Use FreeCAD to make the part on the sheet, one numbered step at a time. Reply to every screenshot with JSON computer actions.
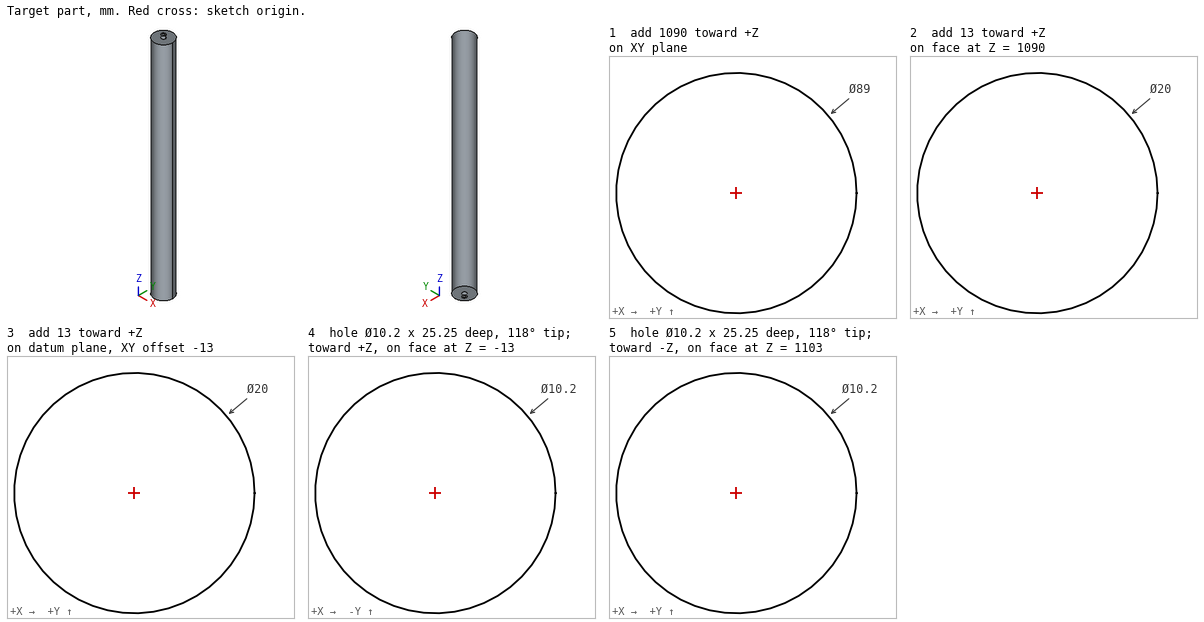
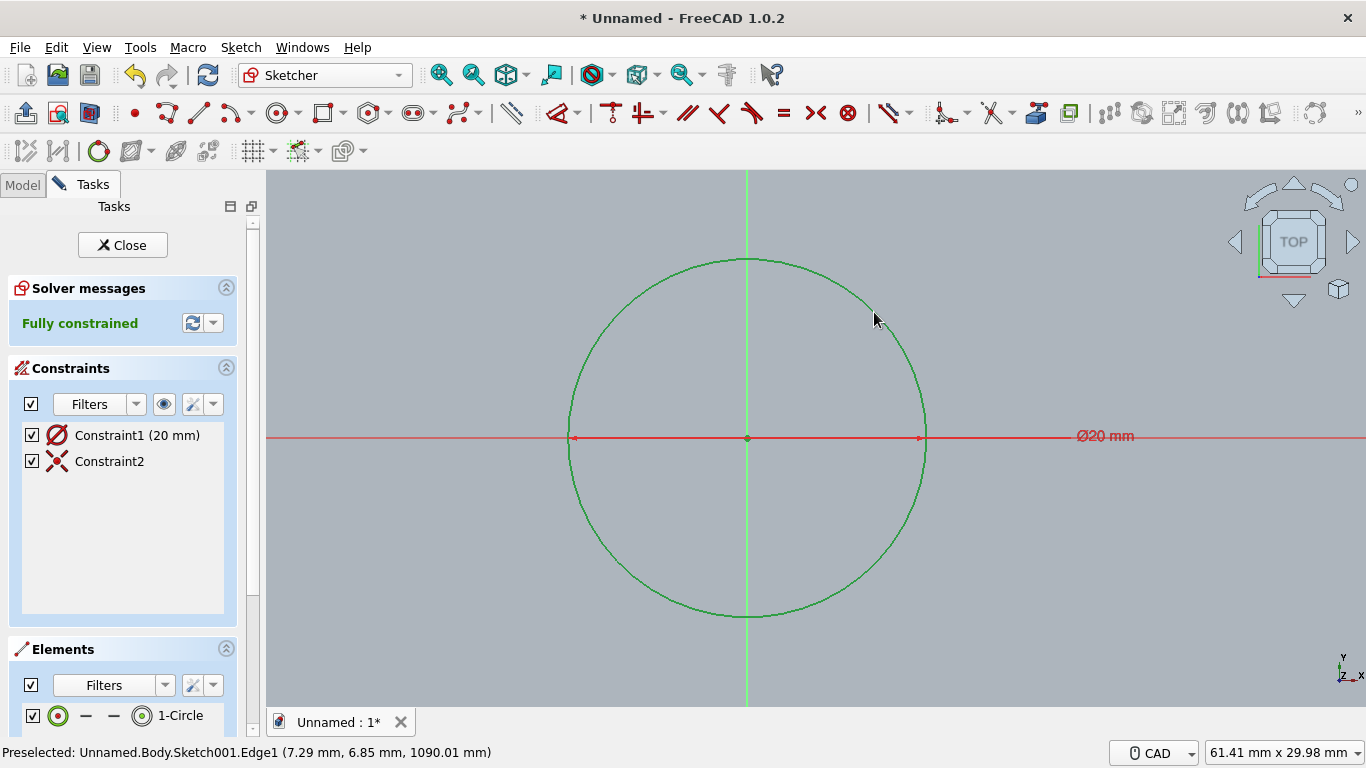
{"action": "left_click", "coordinate": [123, 245]}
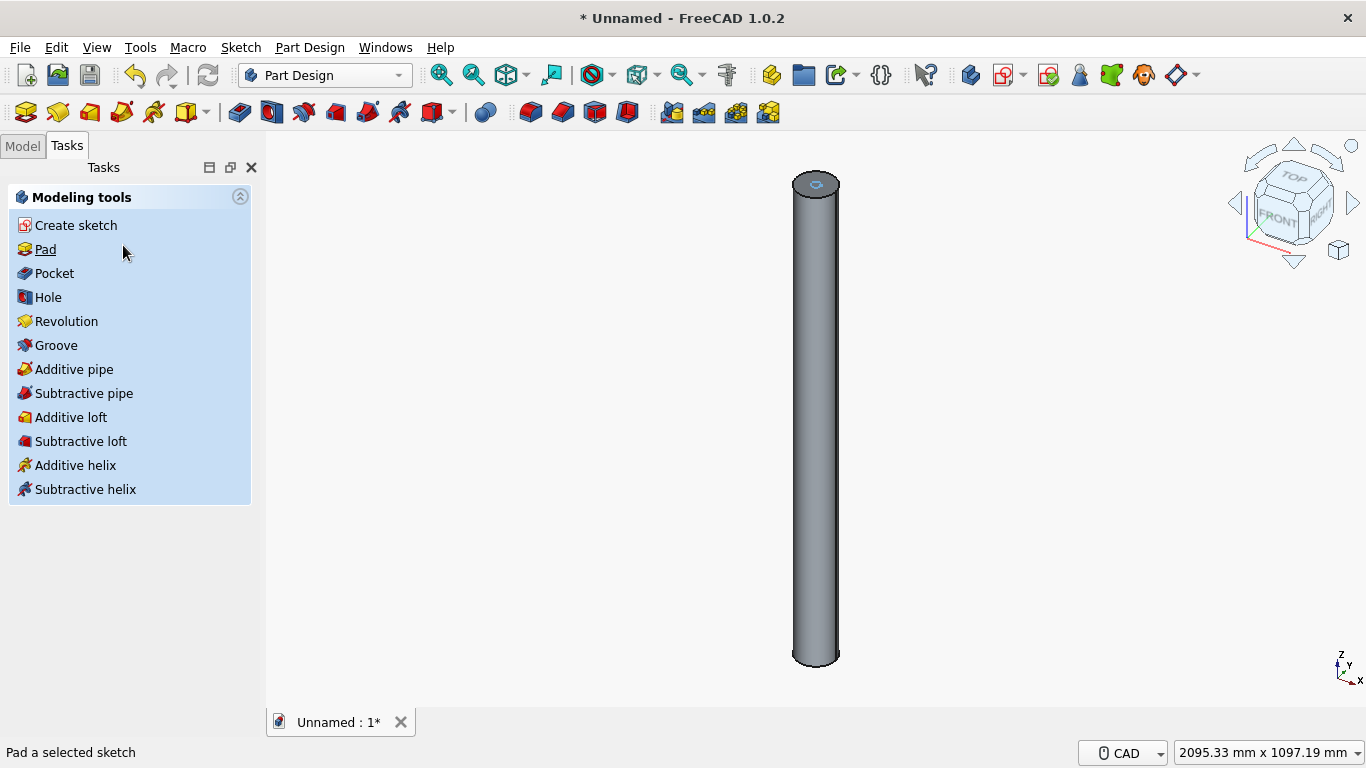
{"action": "left_click", "coordinate": [26, 112]}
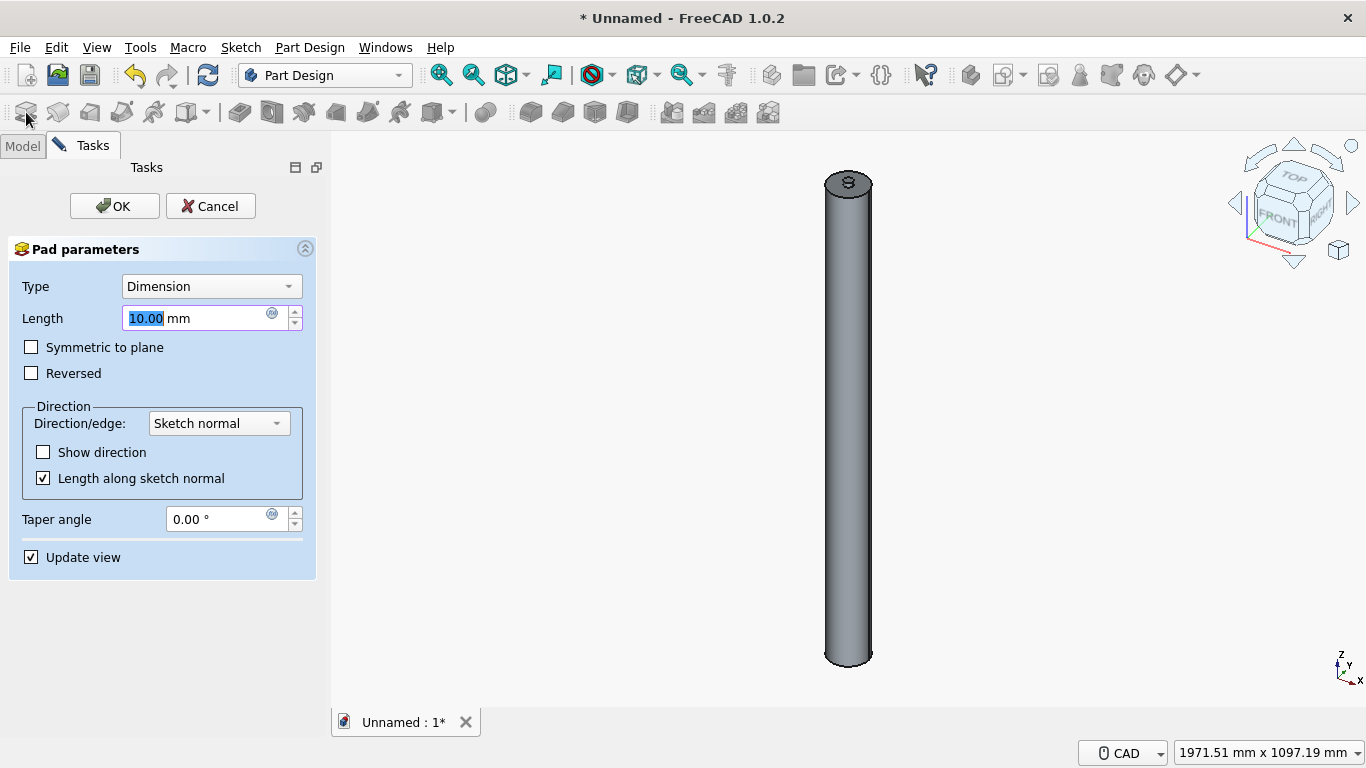
{"action": "type", "text": "13"}
{"action": "key", "text": "Tab"}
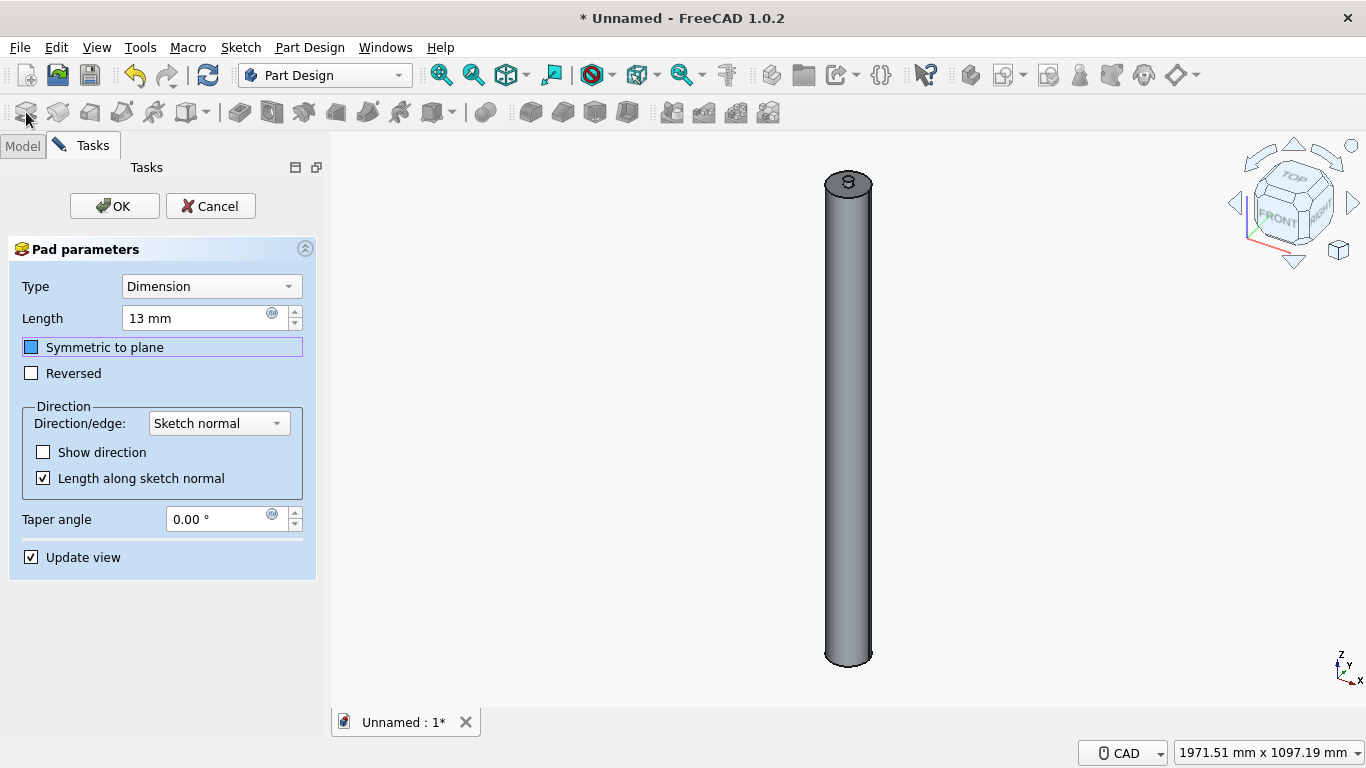
{"action": "left_click", "coordinate": [115, 206]}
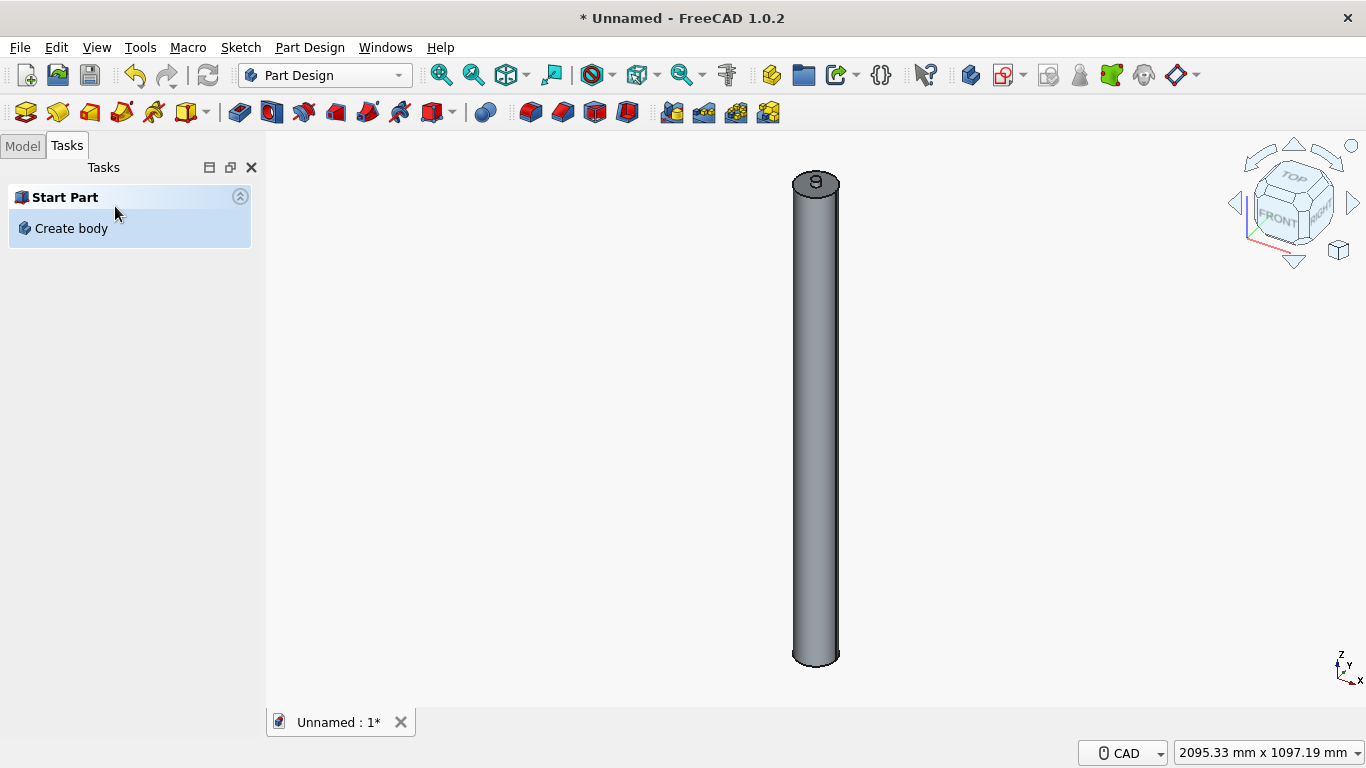
{"action": "left_click", "coordinate": [23, 145]}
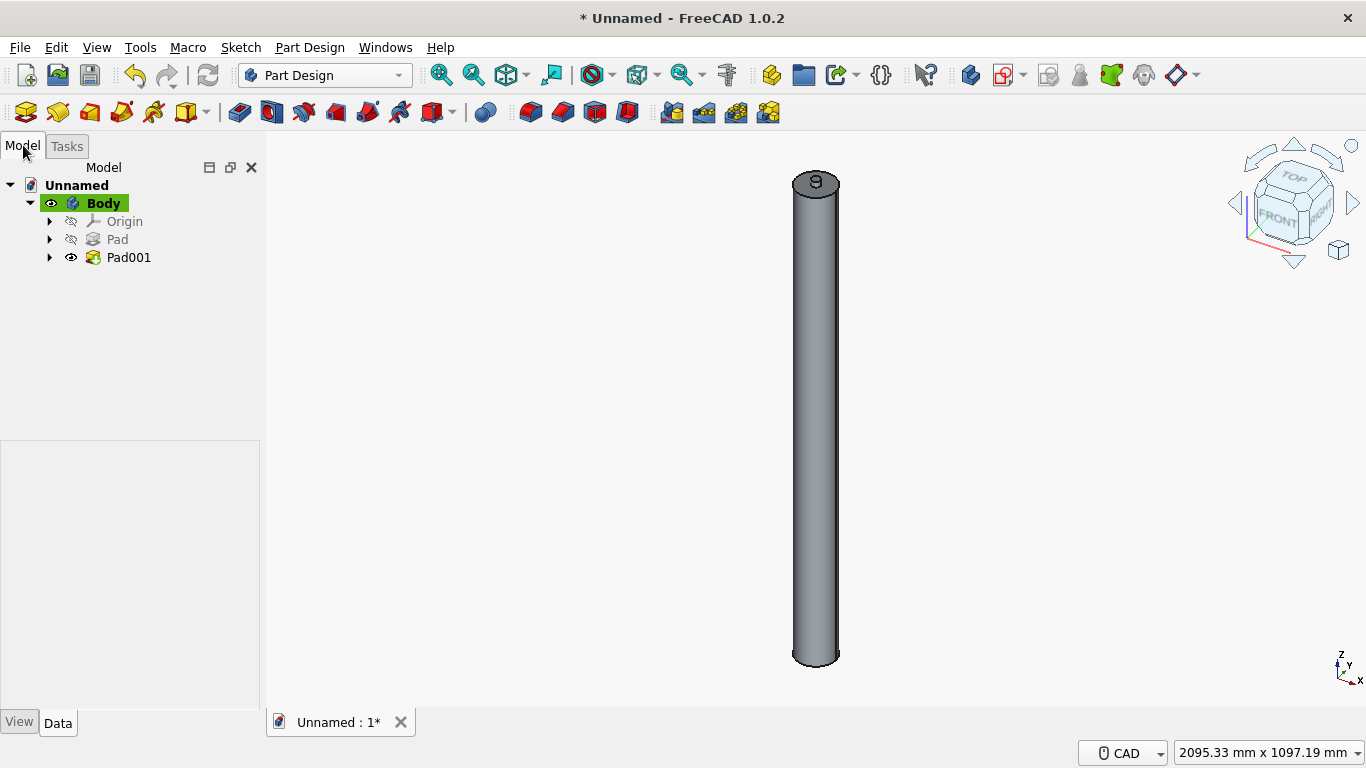
{"action": "left_click", "coordinate": [50, 221]}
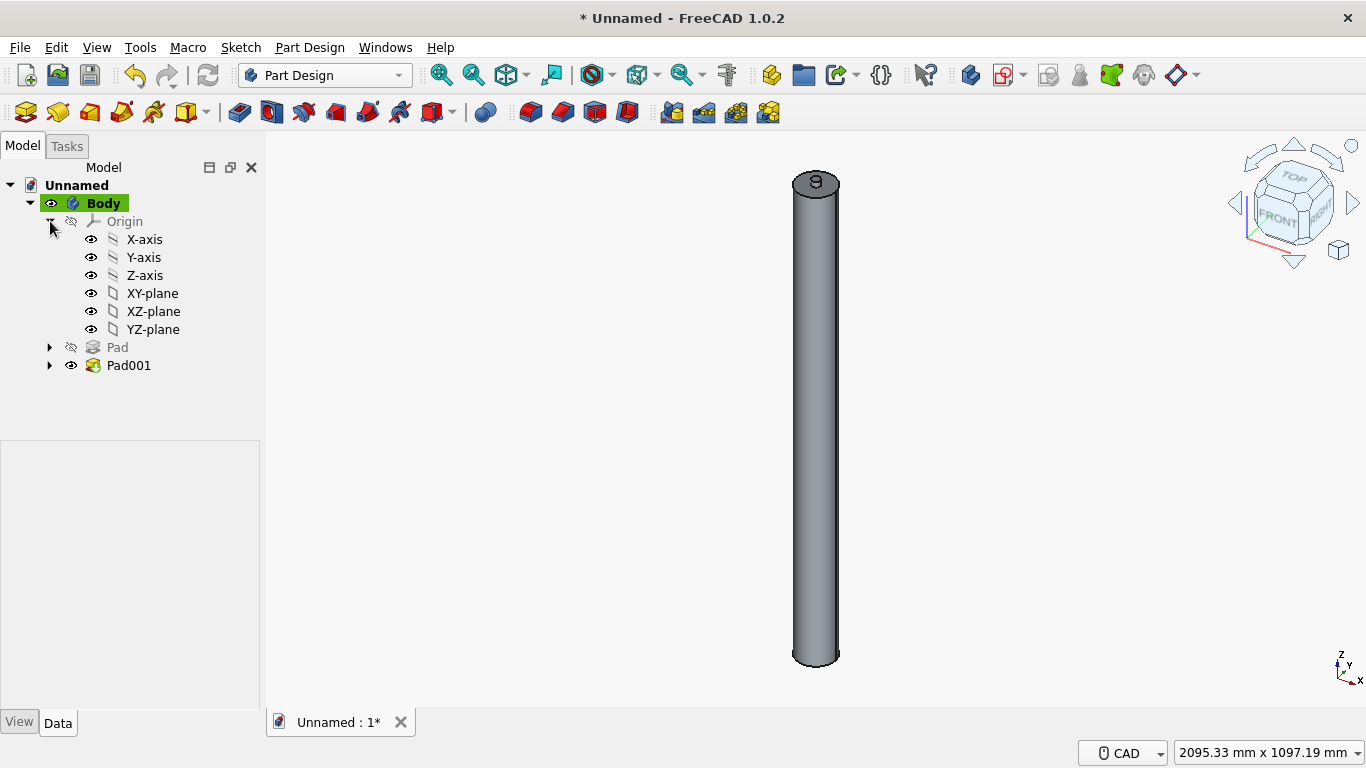
{"action": "left_click", "coordinate": [136, 293]}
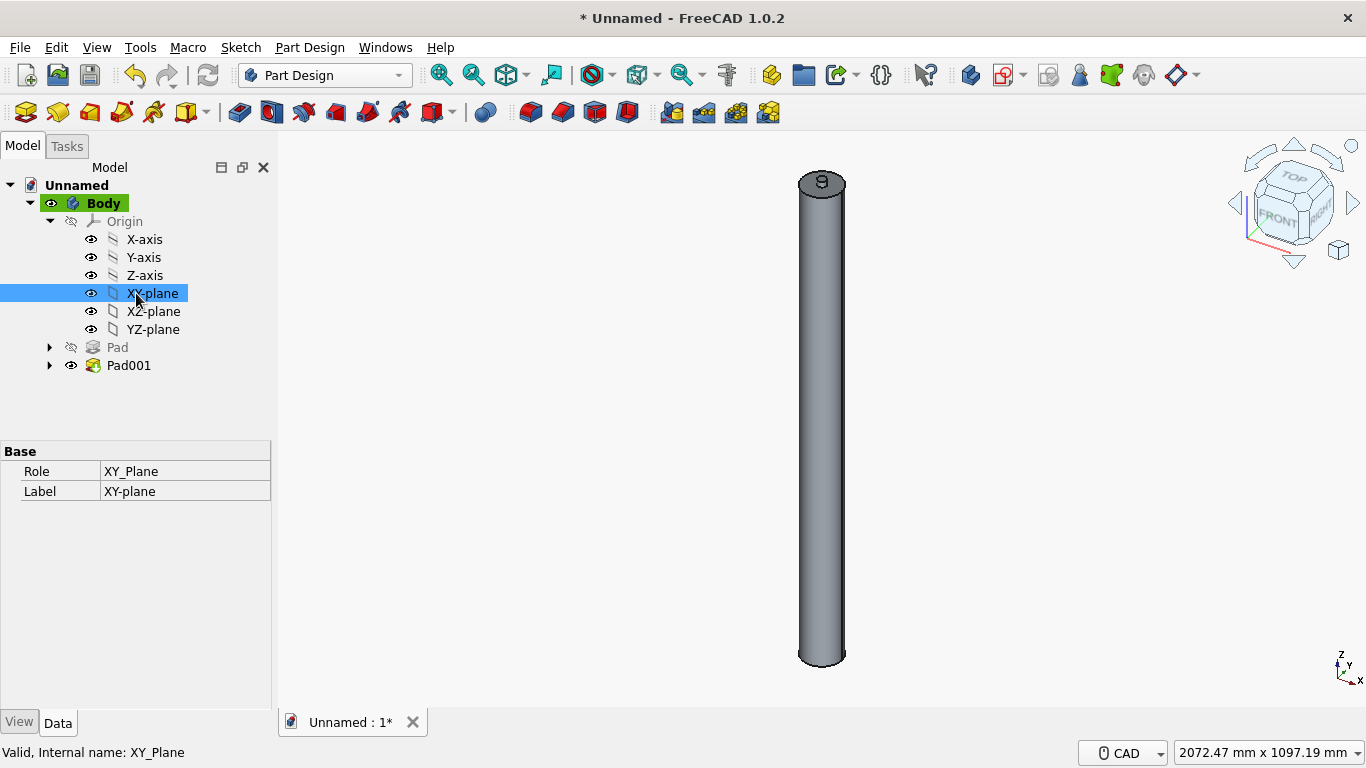
{"action": "left_click", "coordinate": [1176, 76]}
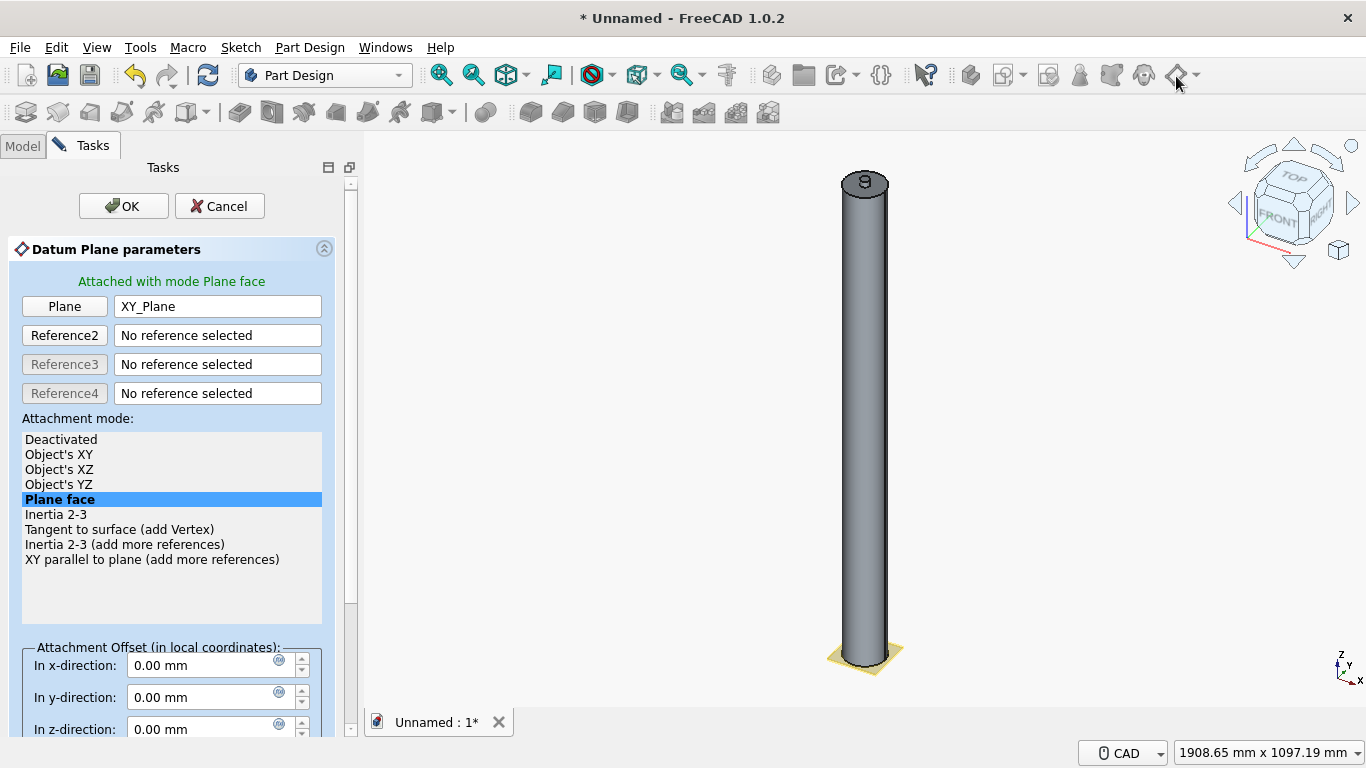
{"action": "scroll", "coordinate": [351, 456], "scroll_direction": "down", "scroll_amount": 2}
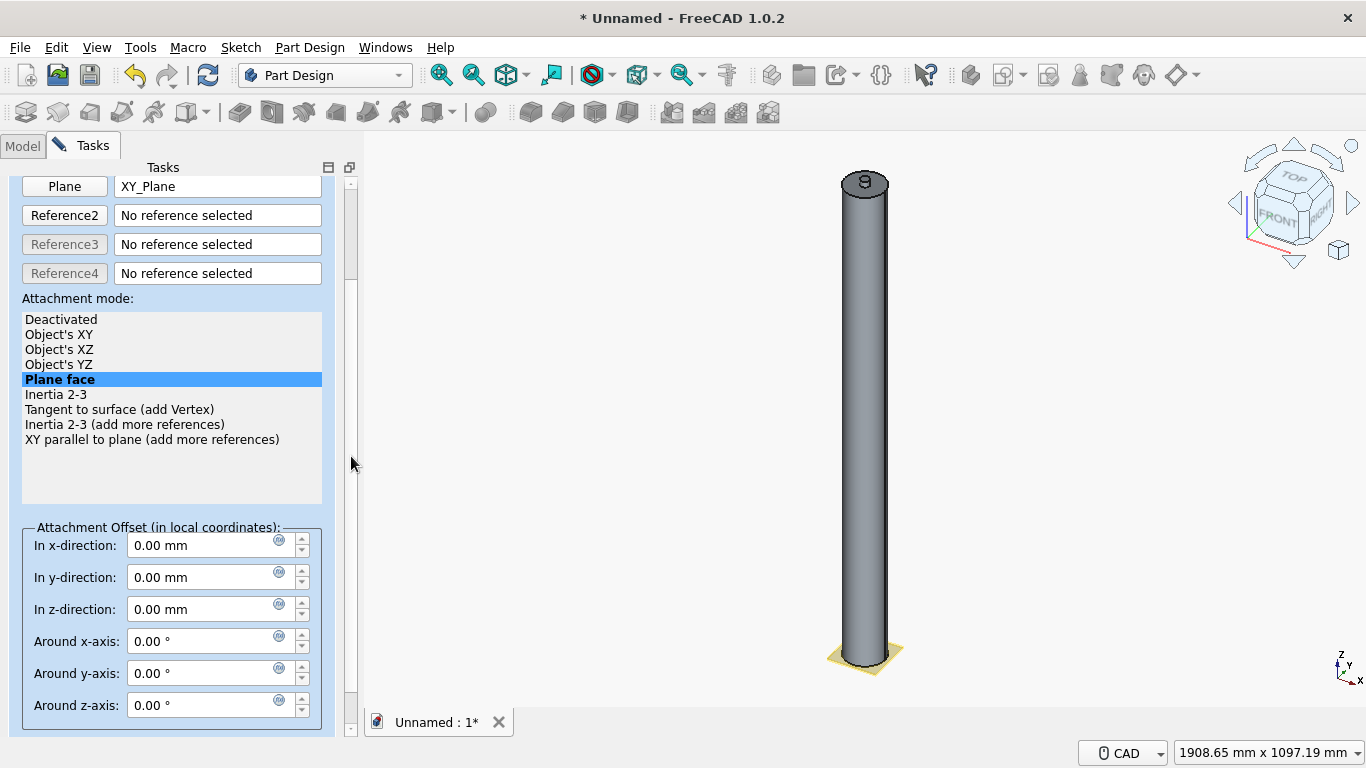
{"action": "triple_click", "coordinate": [210, 609]}